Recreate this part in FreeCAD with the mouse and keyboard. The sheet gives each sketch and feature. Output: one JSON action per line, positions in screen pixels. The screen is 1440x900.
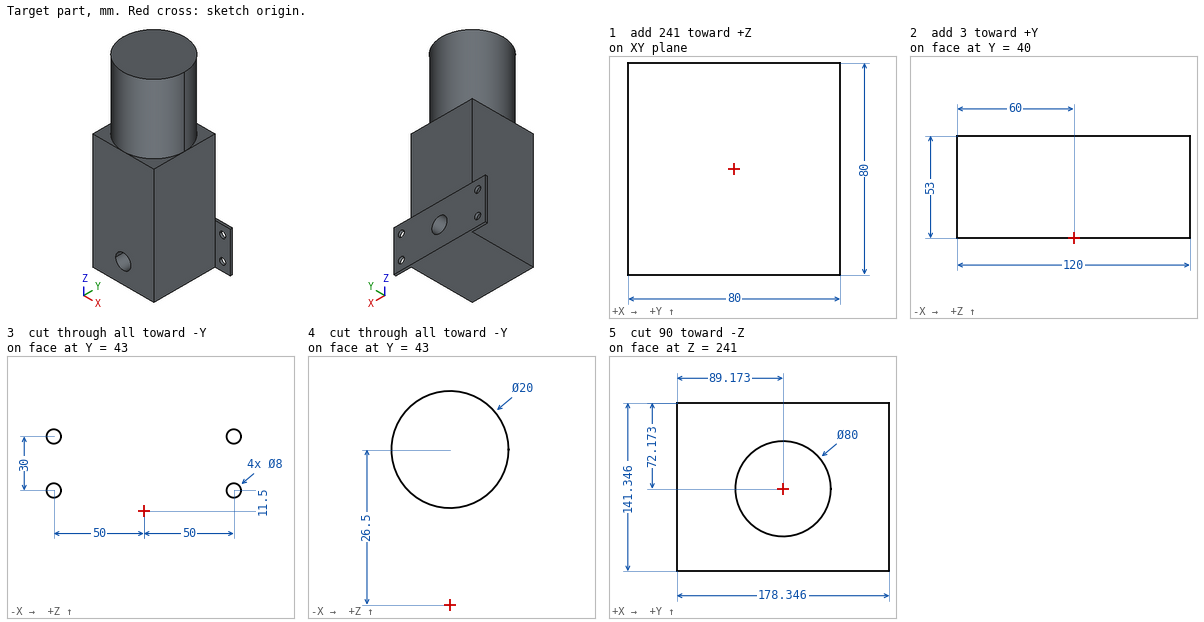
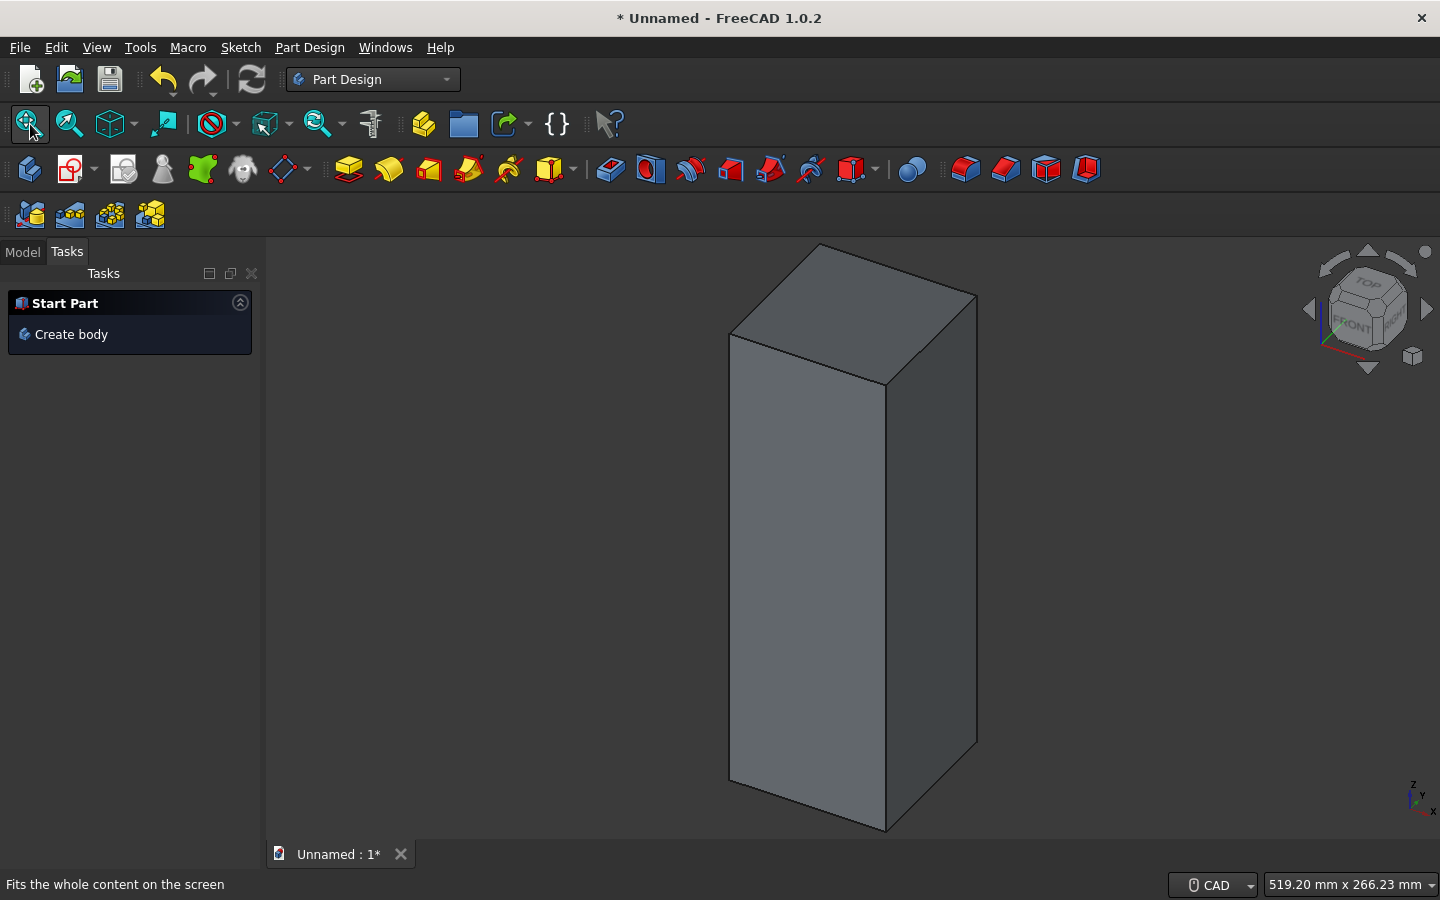
{"action": "key", "text": "4"}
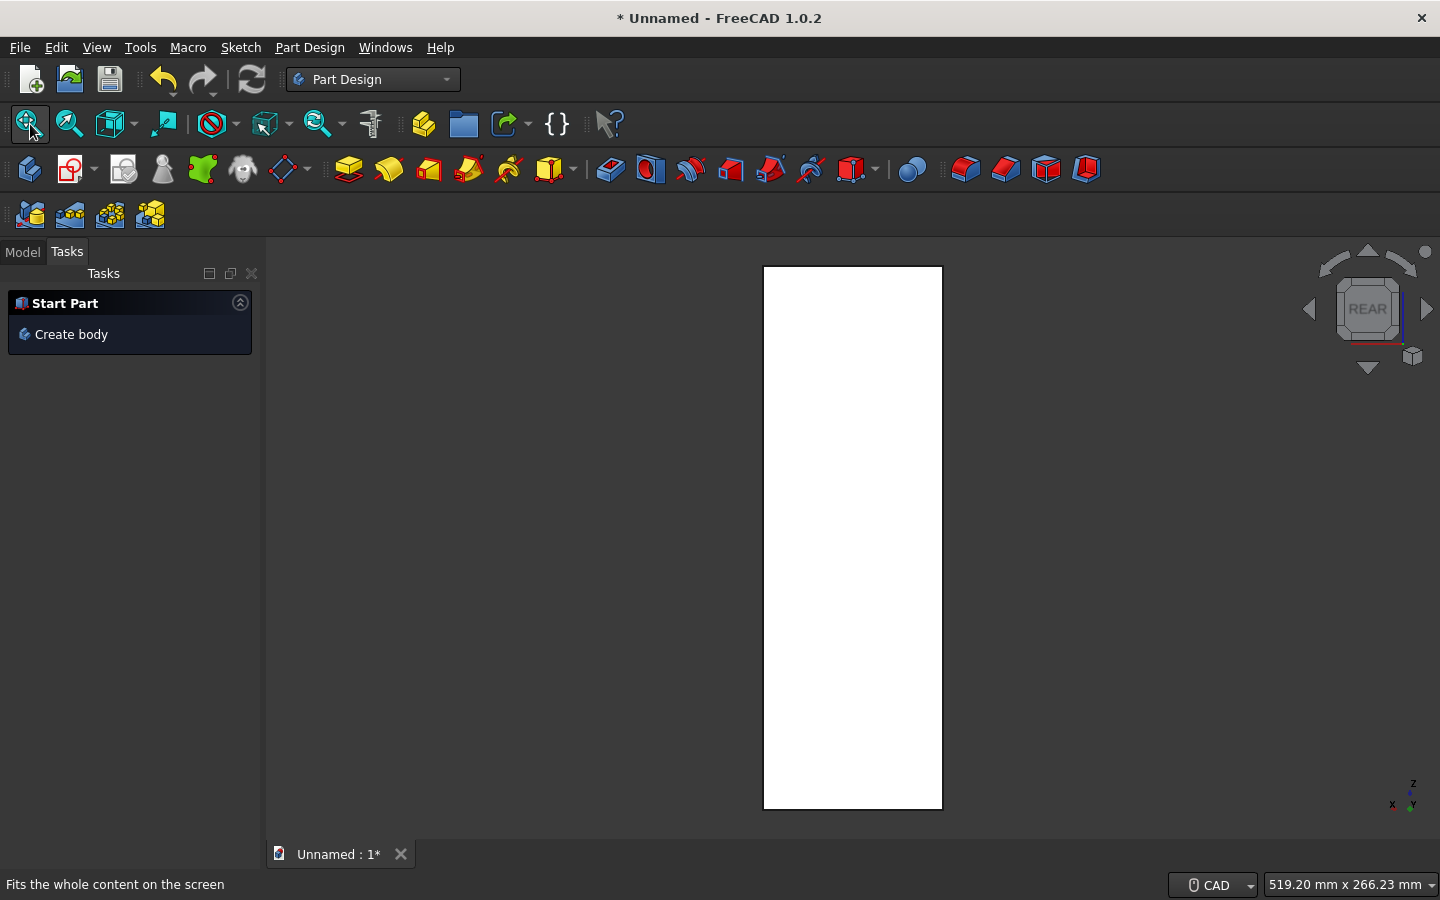
{"action": "left_click", "coordinate": [853, 381]}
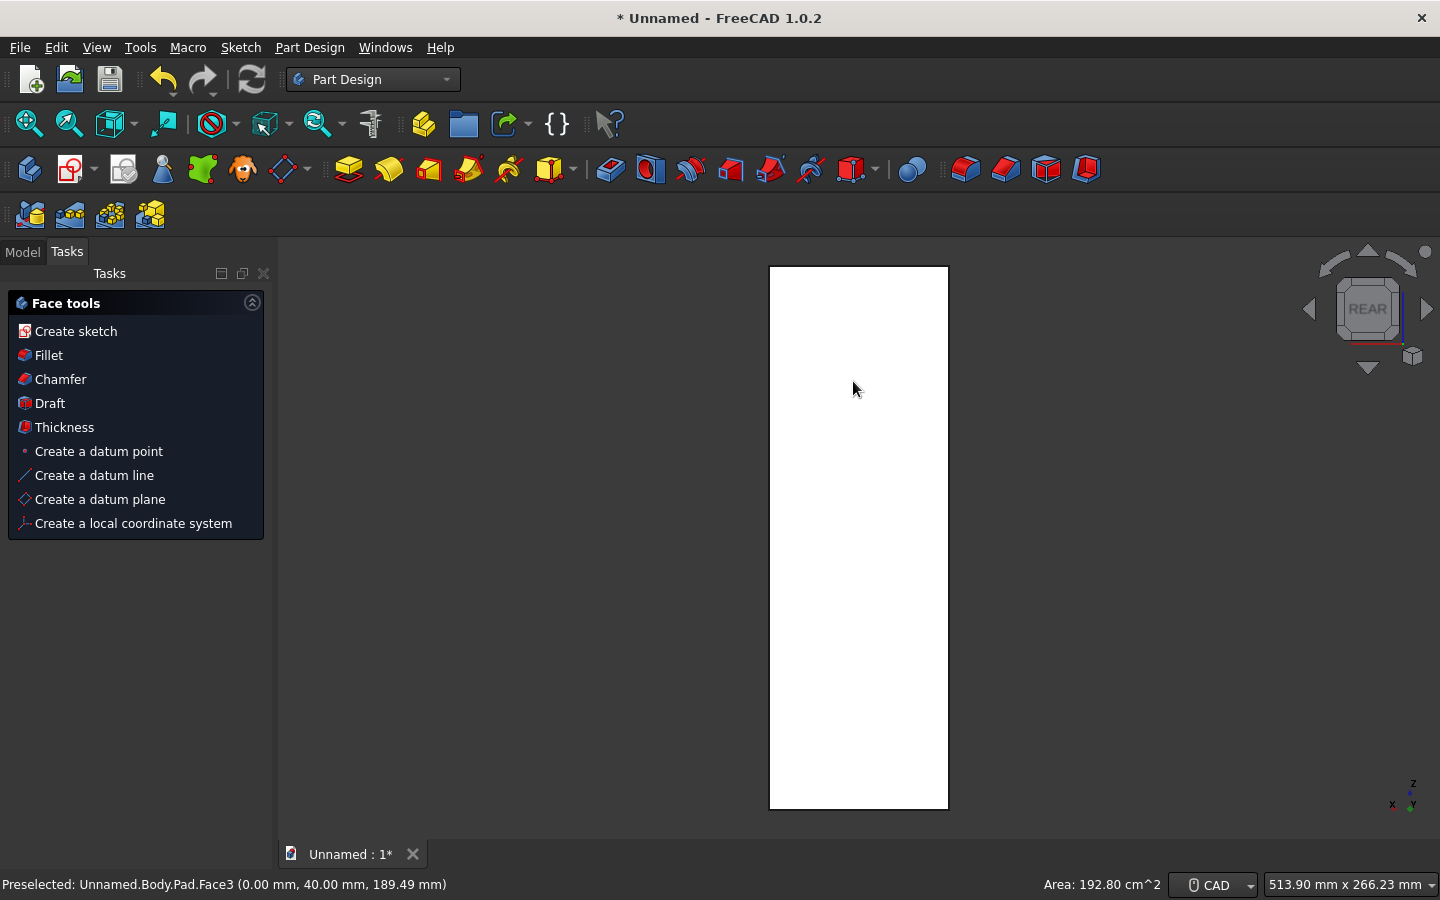
{"action": "left_click", "coordinate": [70, 170]}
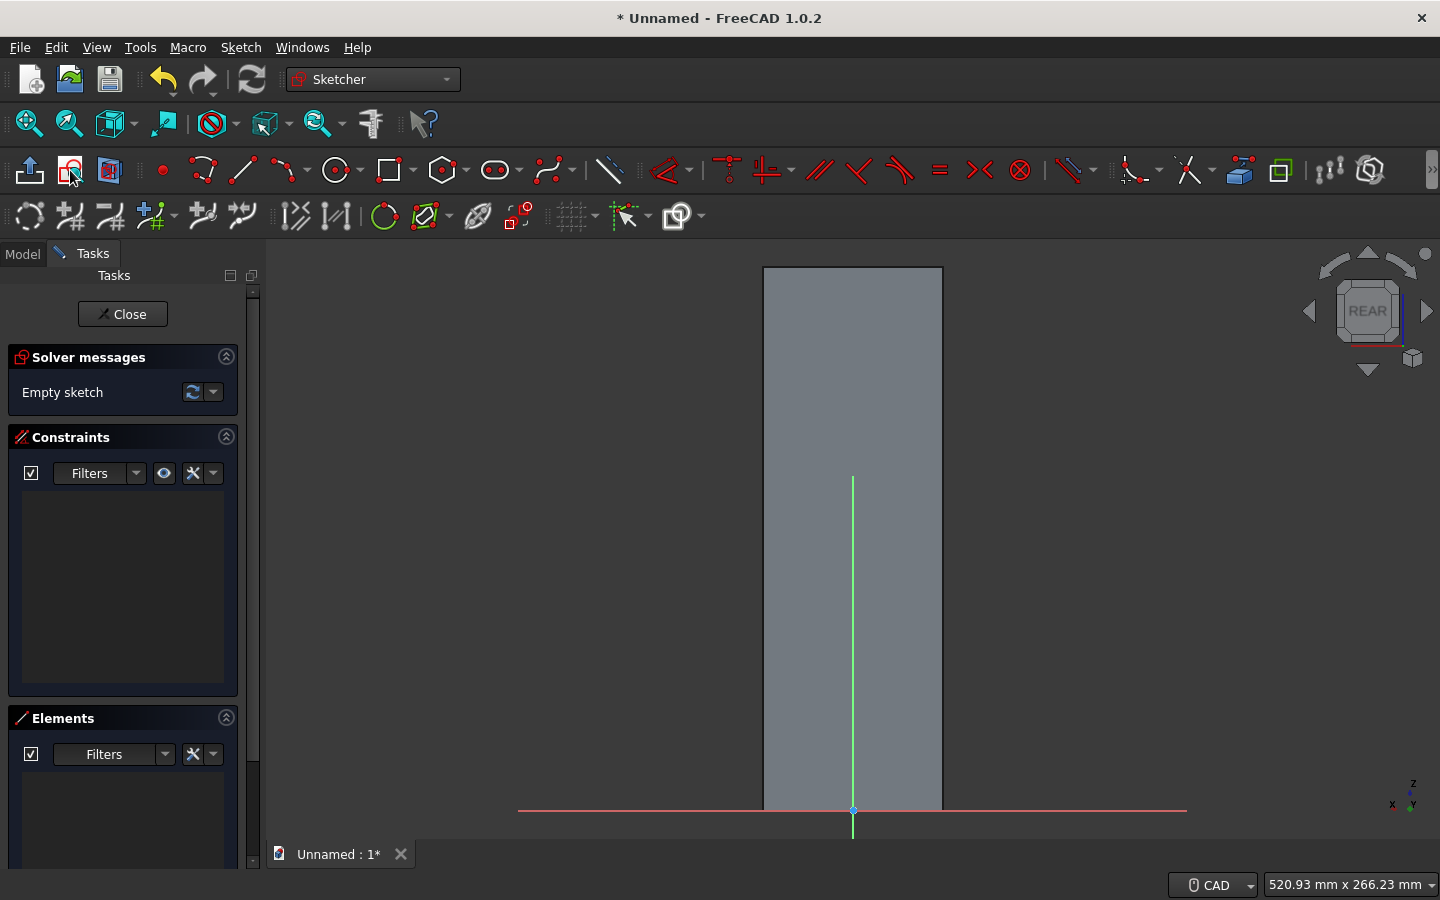
{"action": "scroll", "coordinate": [784, 539], "scroll_direction": "down", "scroll_amount": 5}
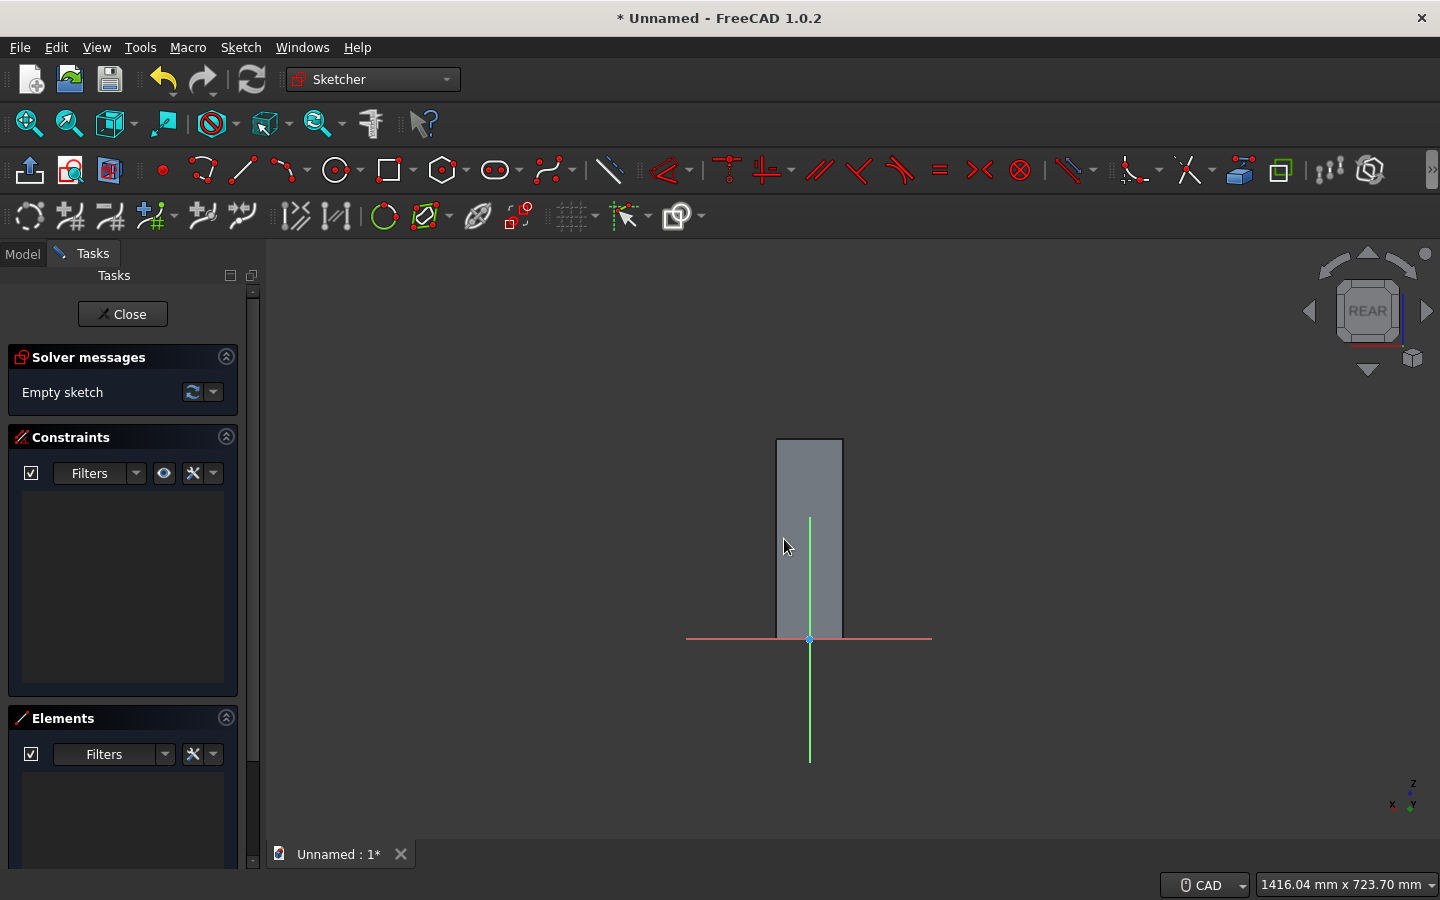
{"action": "scroll", "coordinate": [814, 629], "scroll_direction": "up", "scroll_amount": 10}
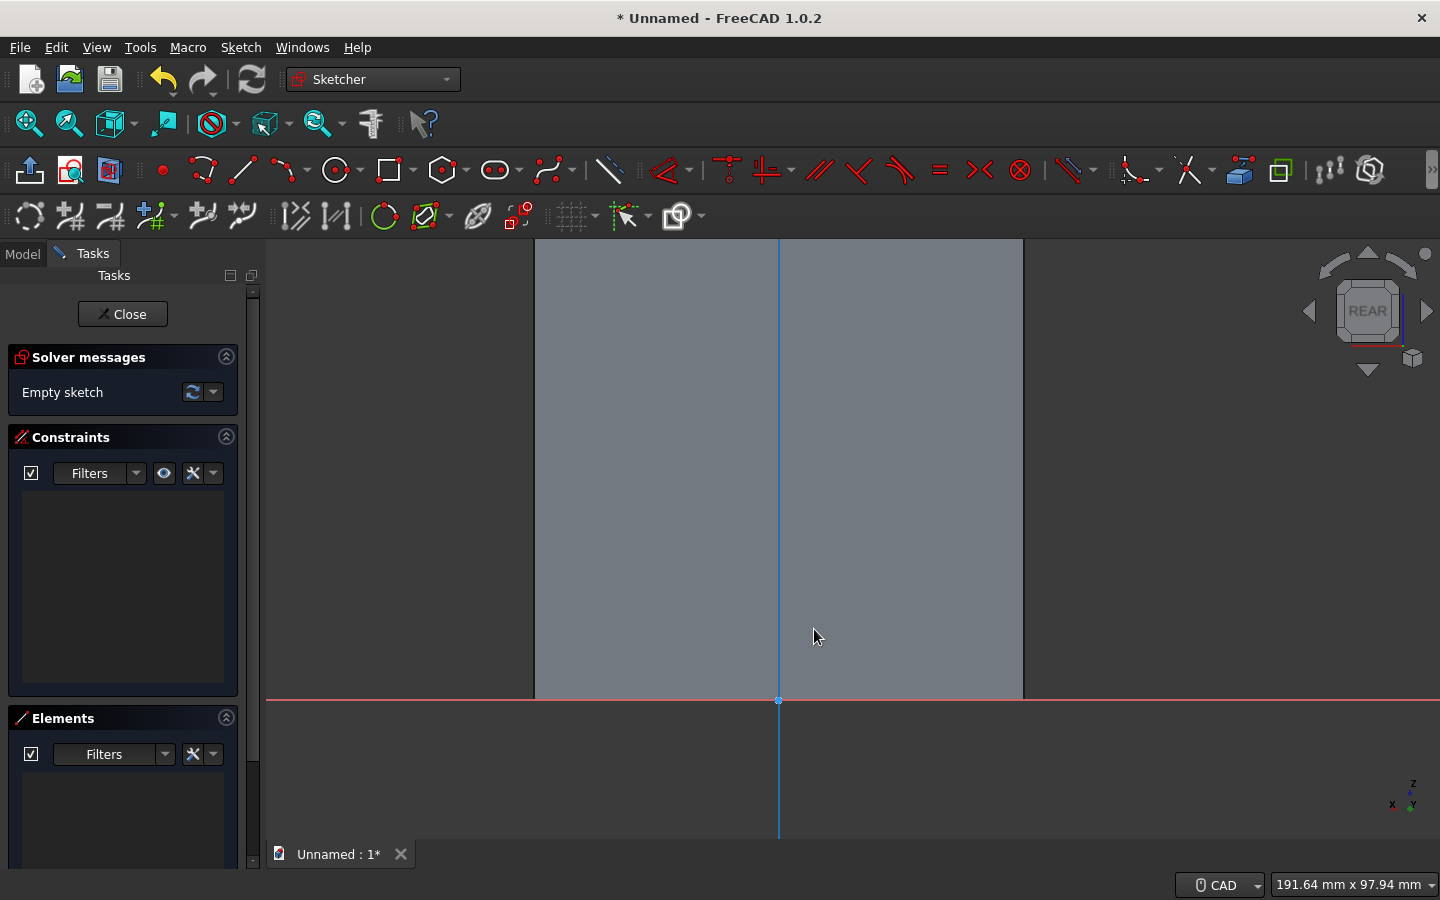
{"action": "left_click", "coordinate": [390, 170]}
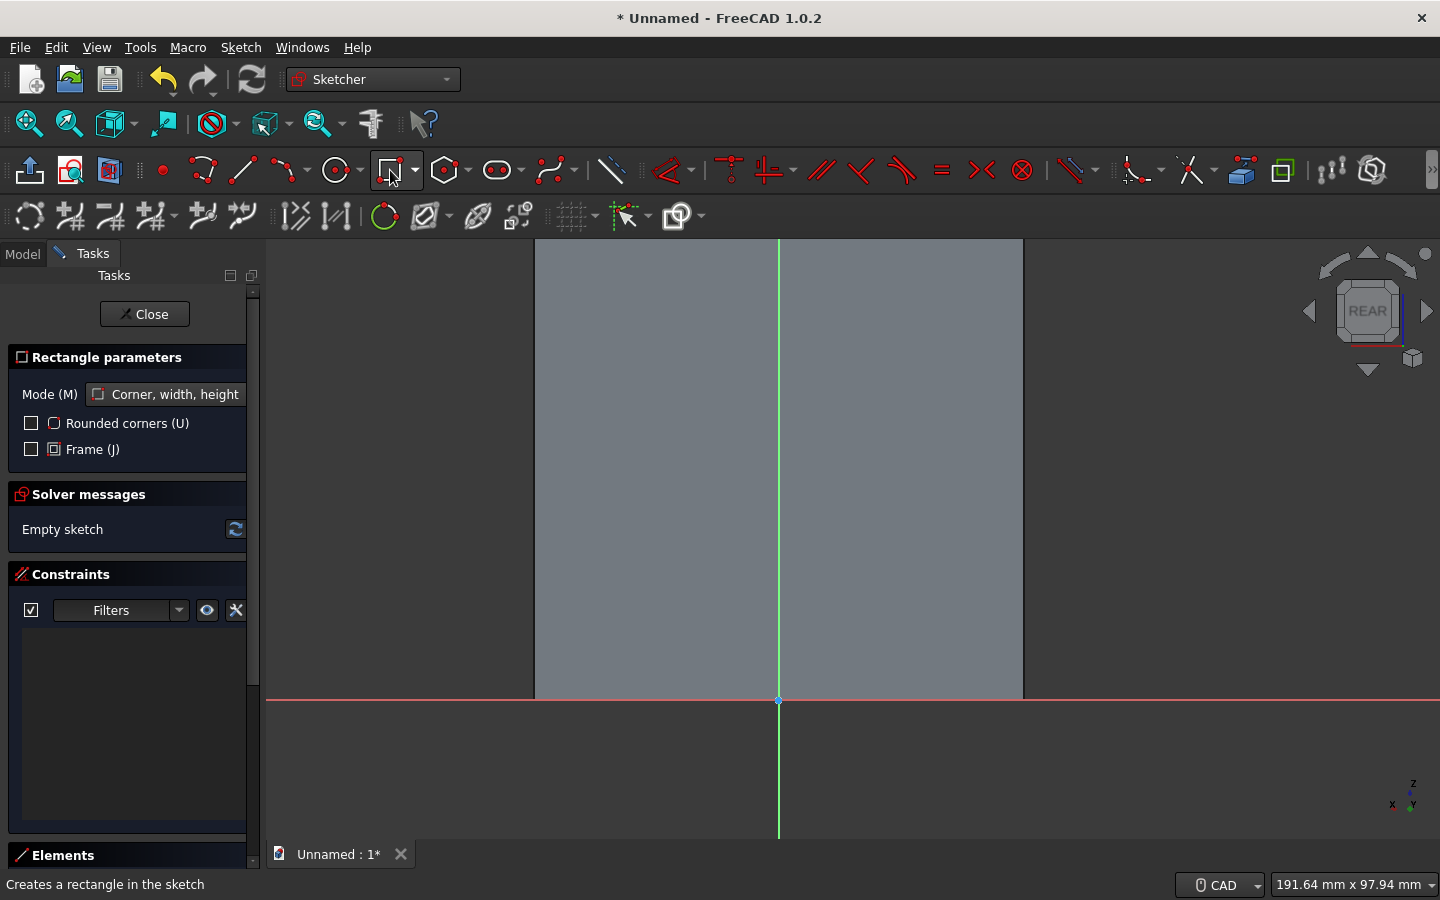
{"action": "left_click", "coordinate": [411, 376]}
{"action": "left_click", "coordinate": [1147, 700]}
{"action": "key", "text": "Escape"}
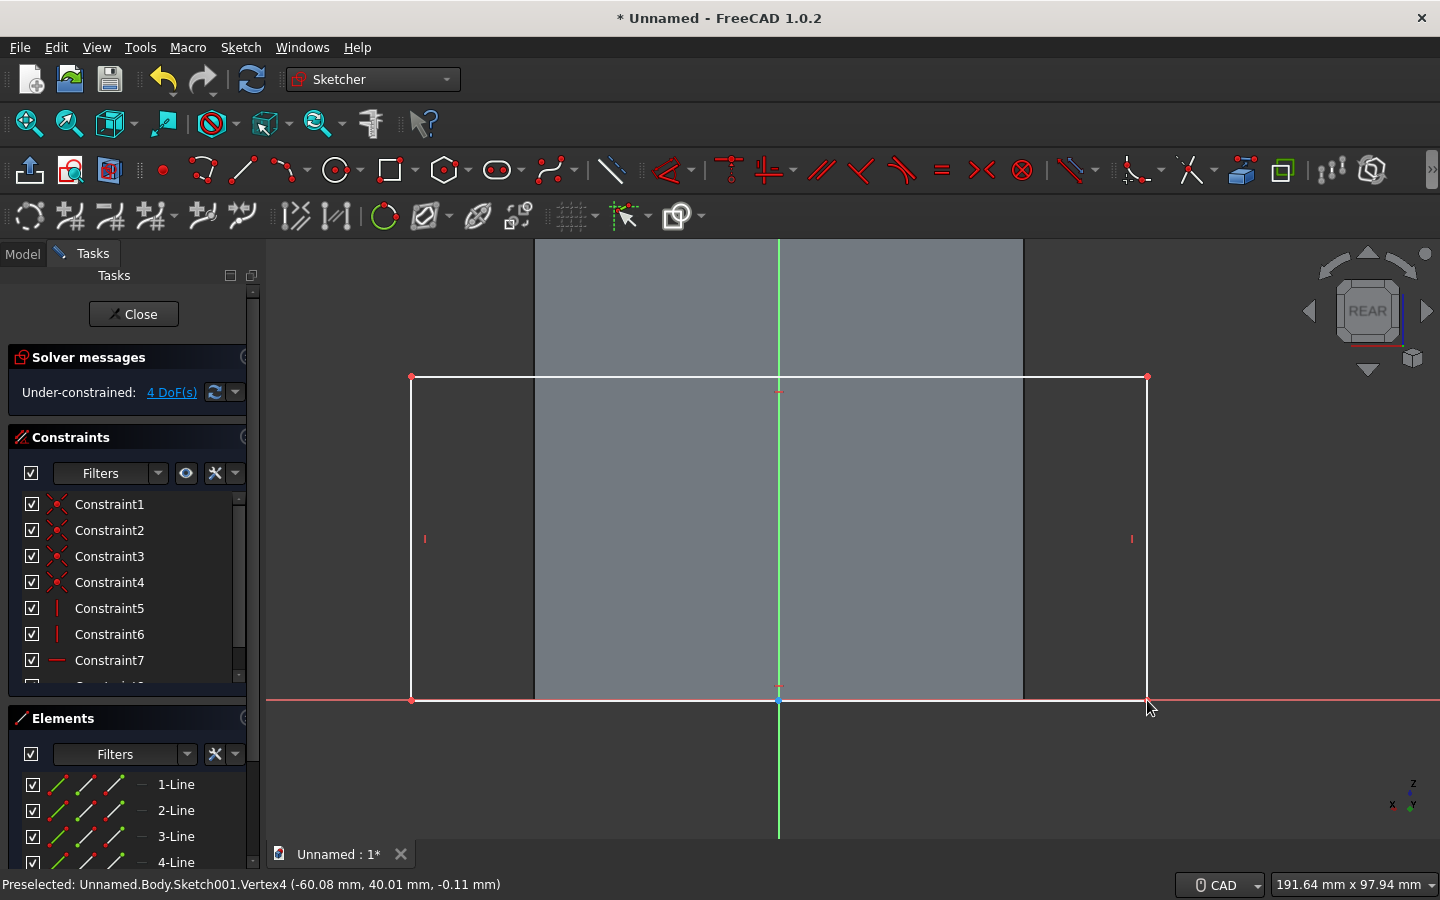
{"action": "left_click", "coordinate": [411, 701]}